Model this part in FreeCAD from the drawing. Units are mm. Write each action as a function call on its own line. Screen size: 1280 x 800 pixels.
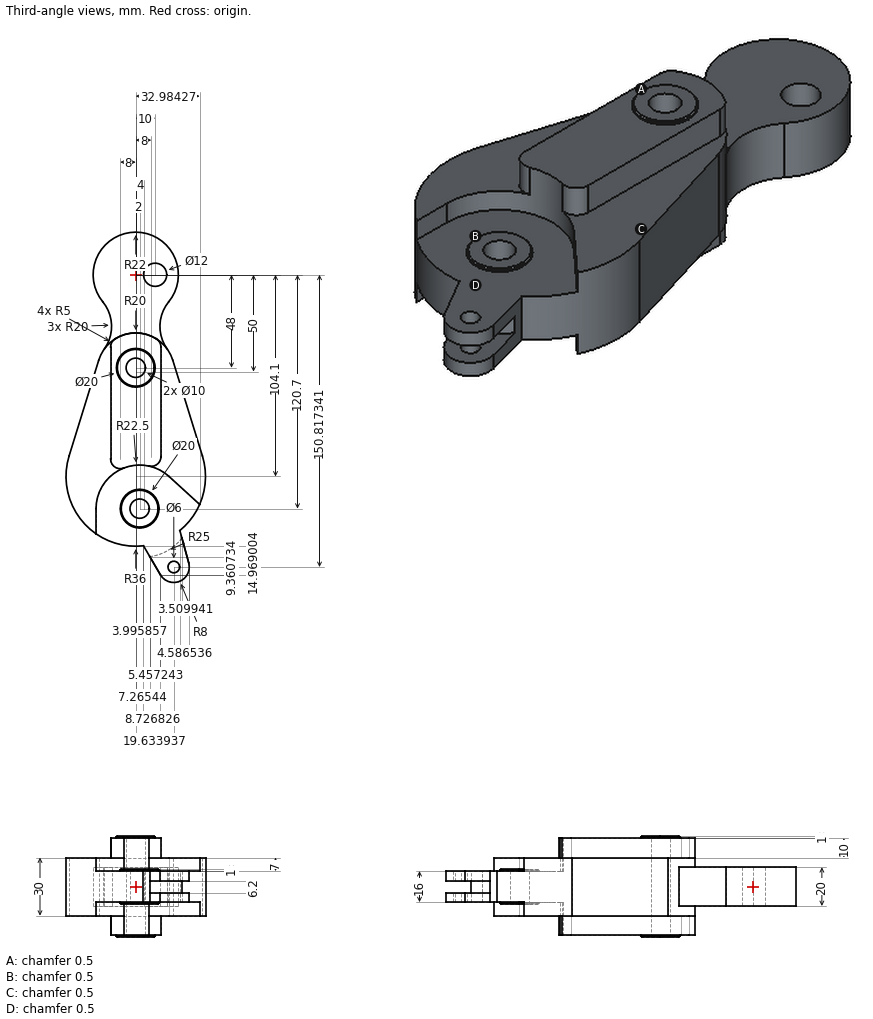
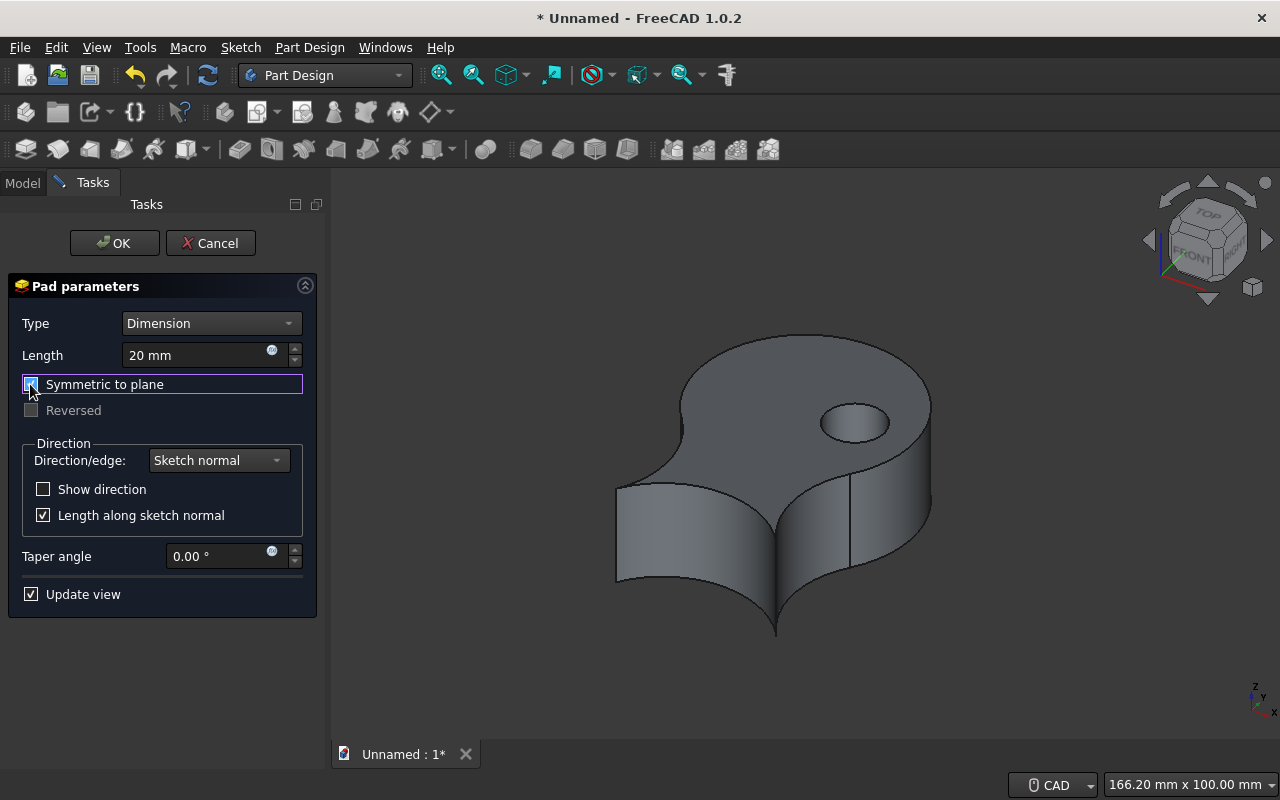
click(115, 243)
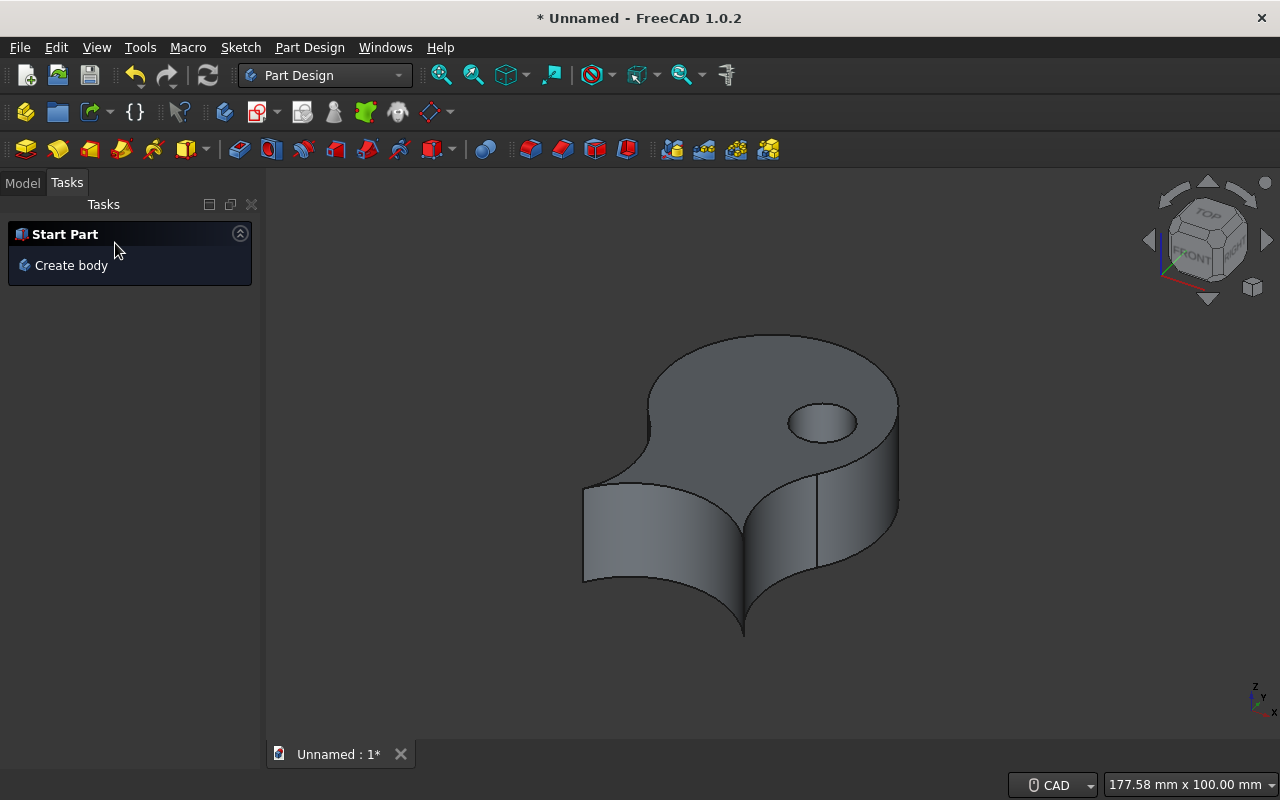
click(258, 112)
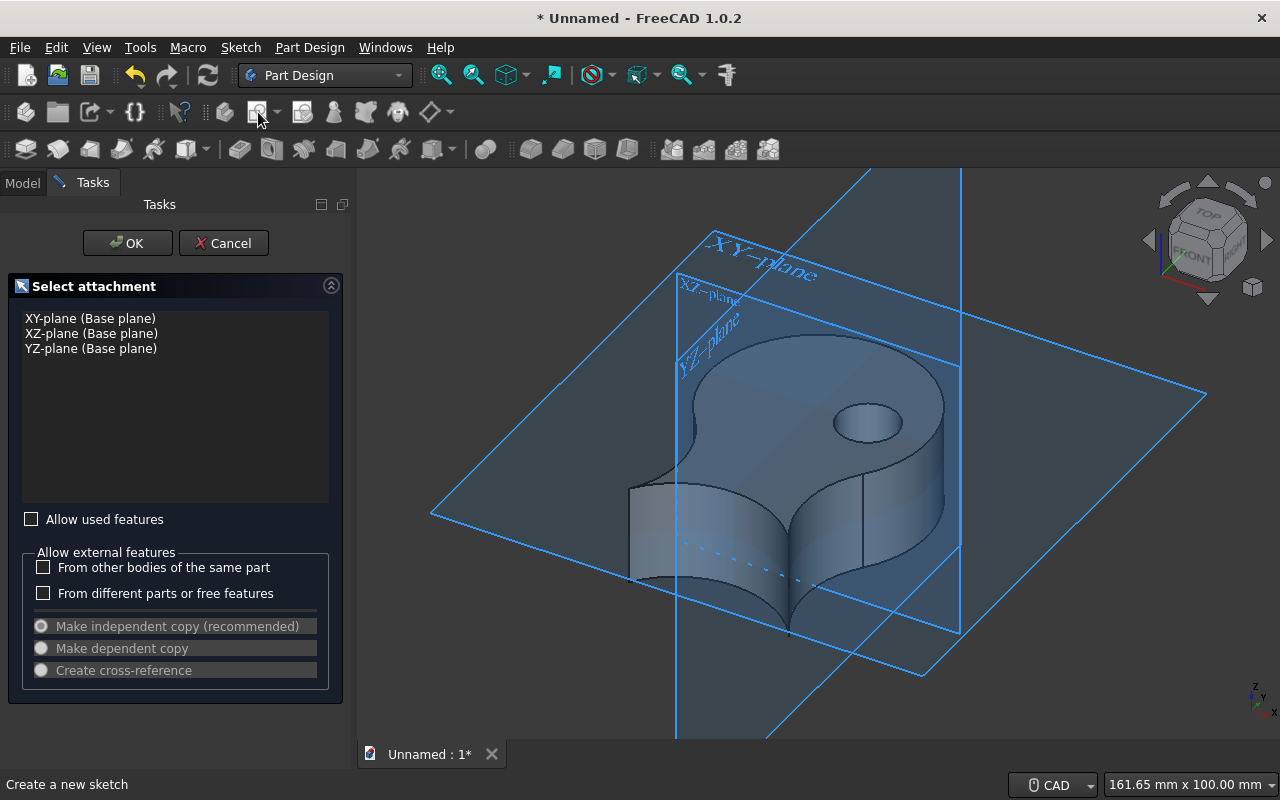
click(82, 318)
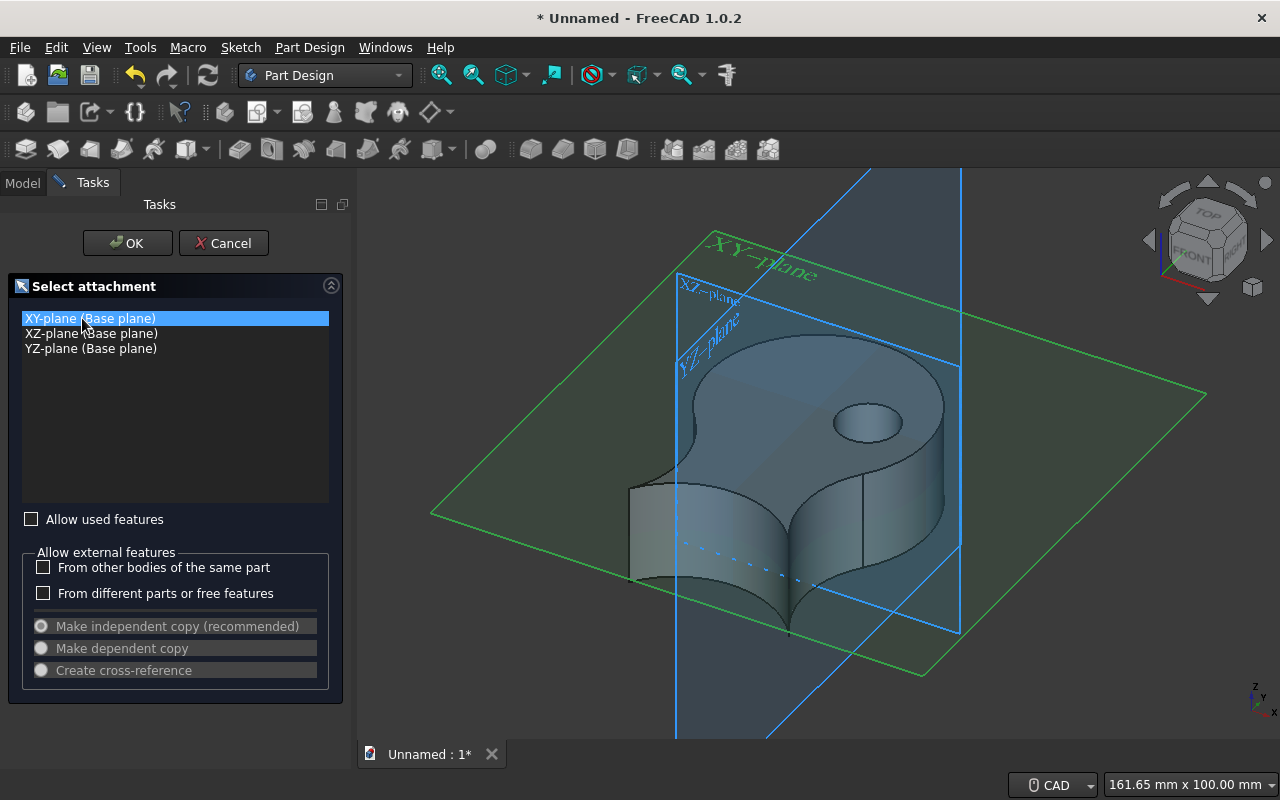
click(128, 243)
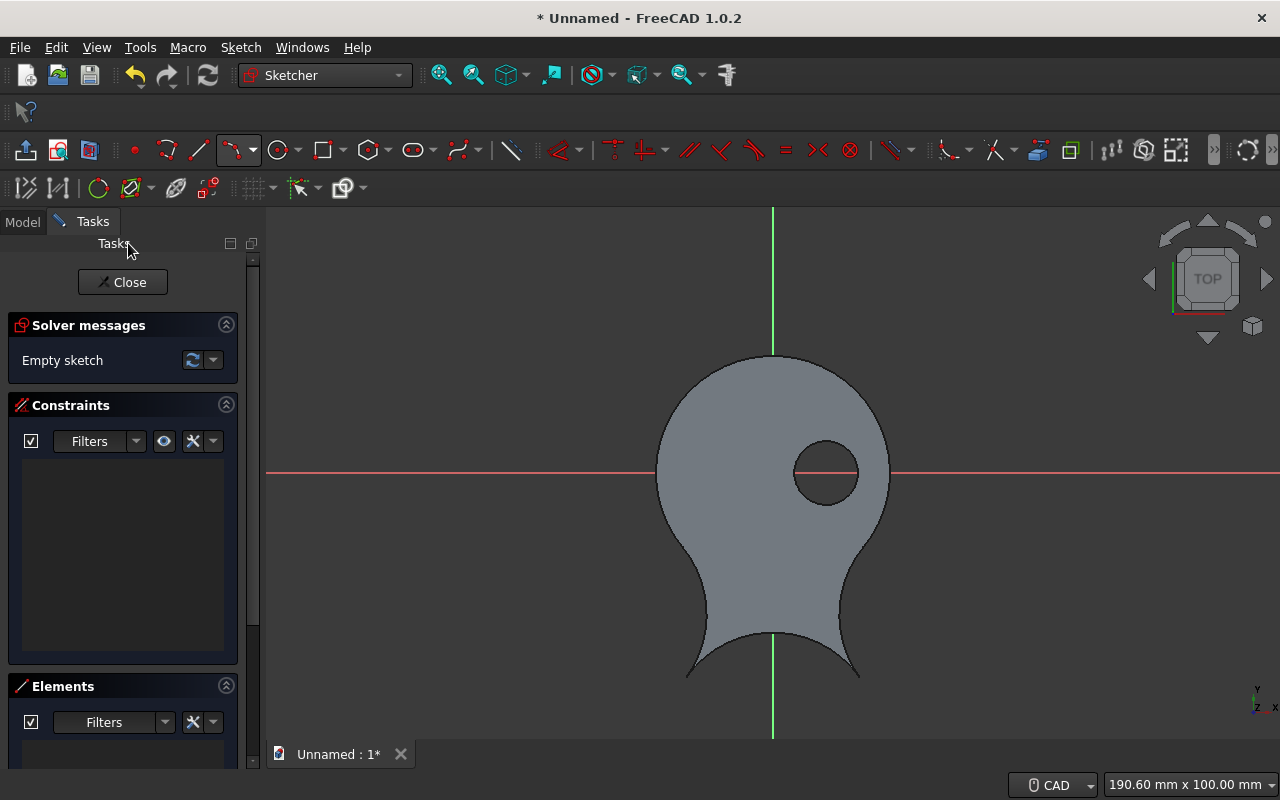
click(90, 150)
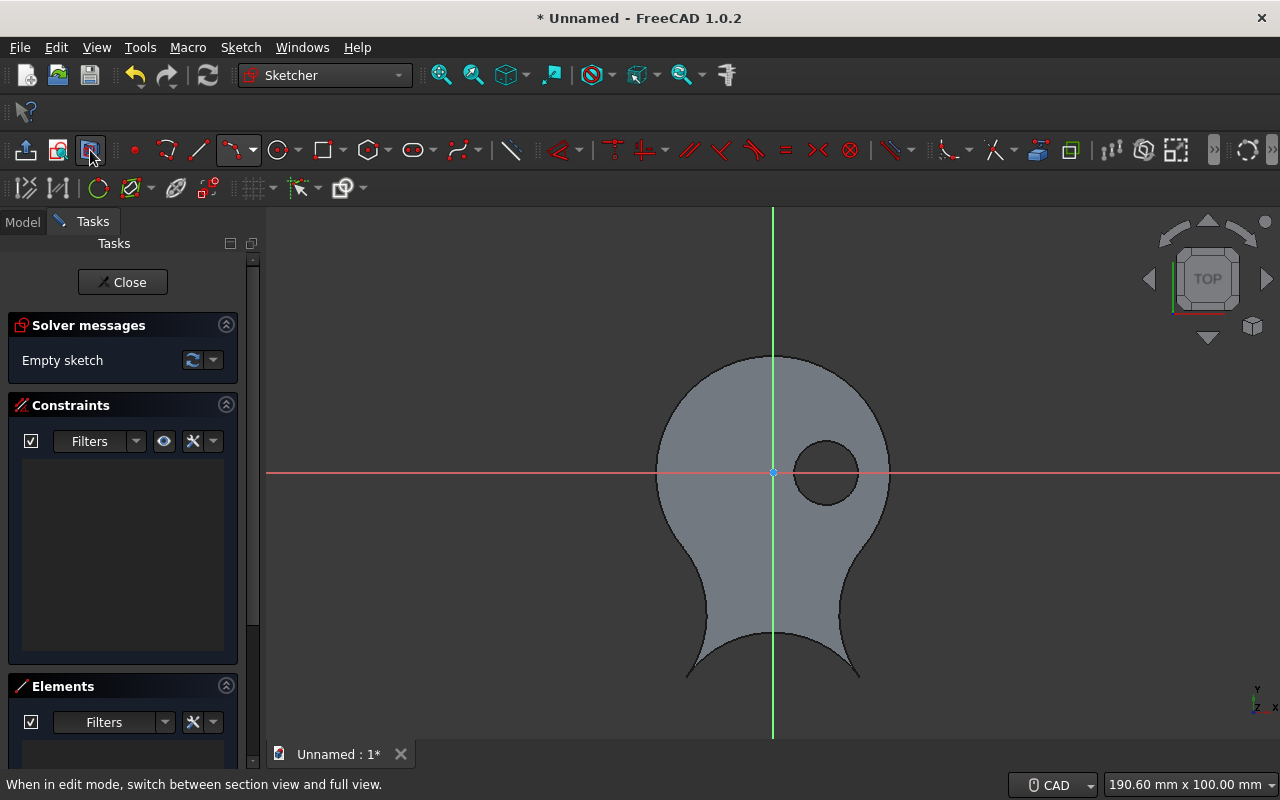
scroll(649, 235, down, 4)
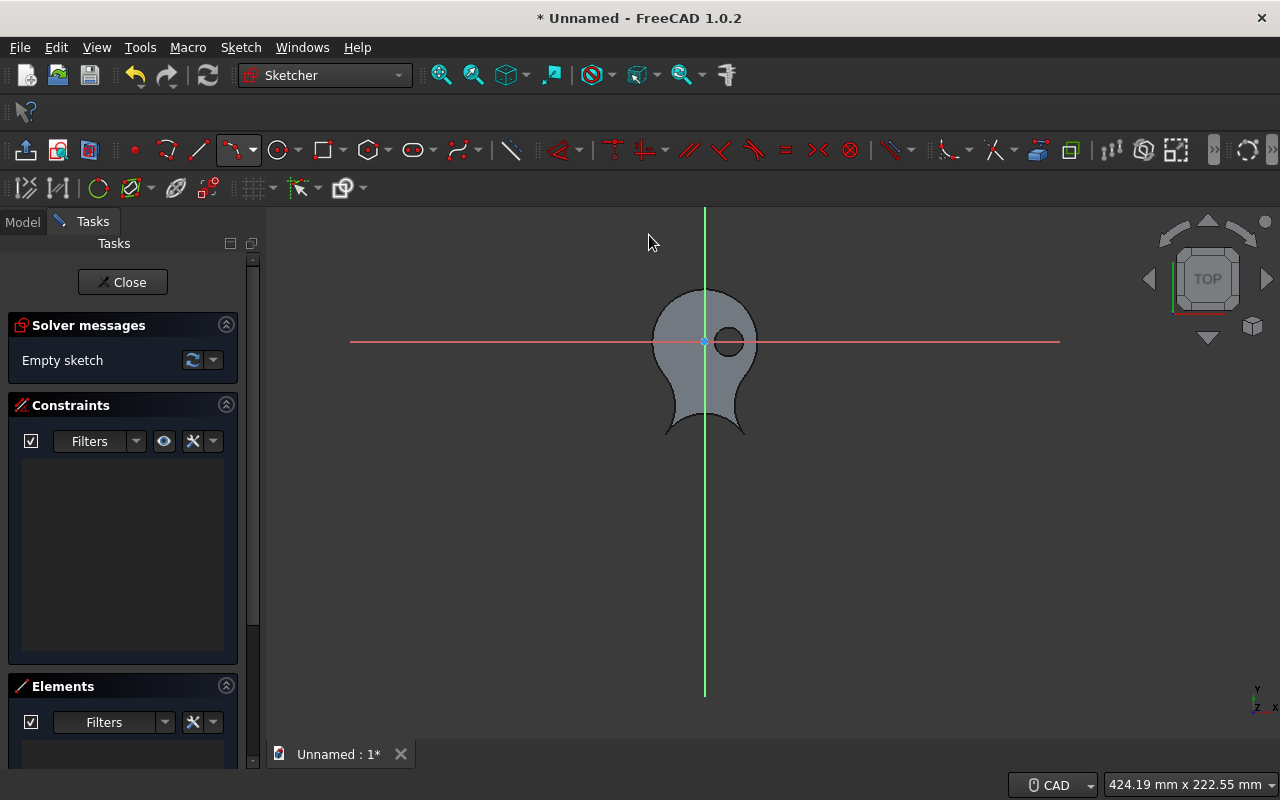
click(200, 150)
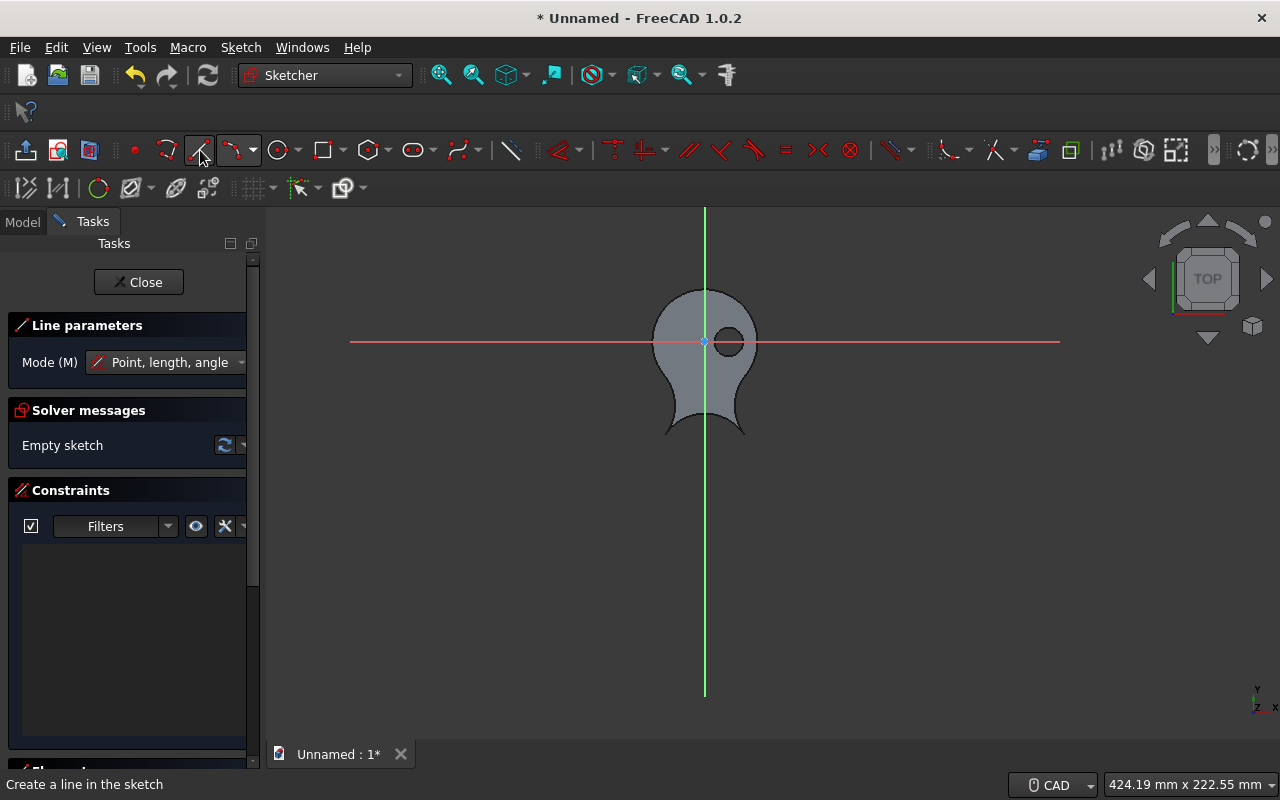
click(659, 447)
click(623, 565)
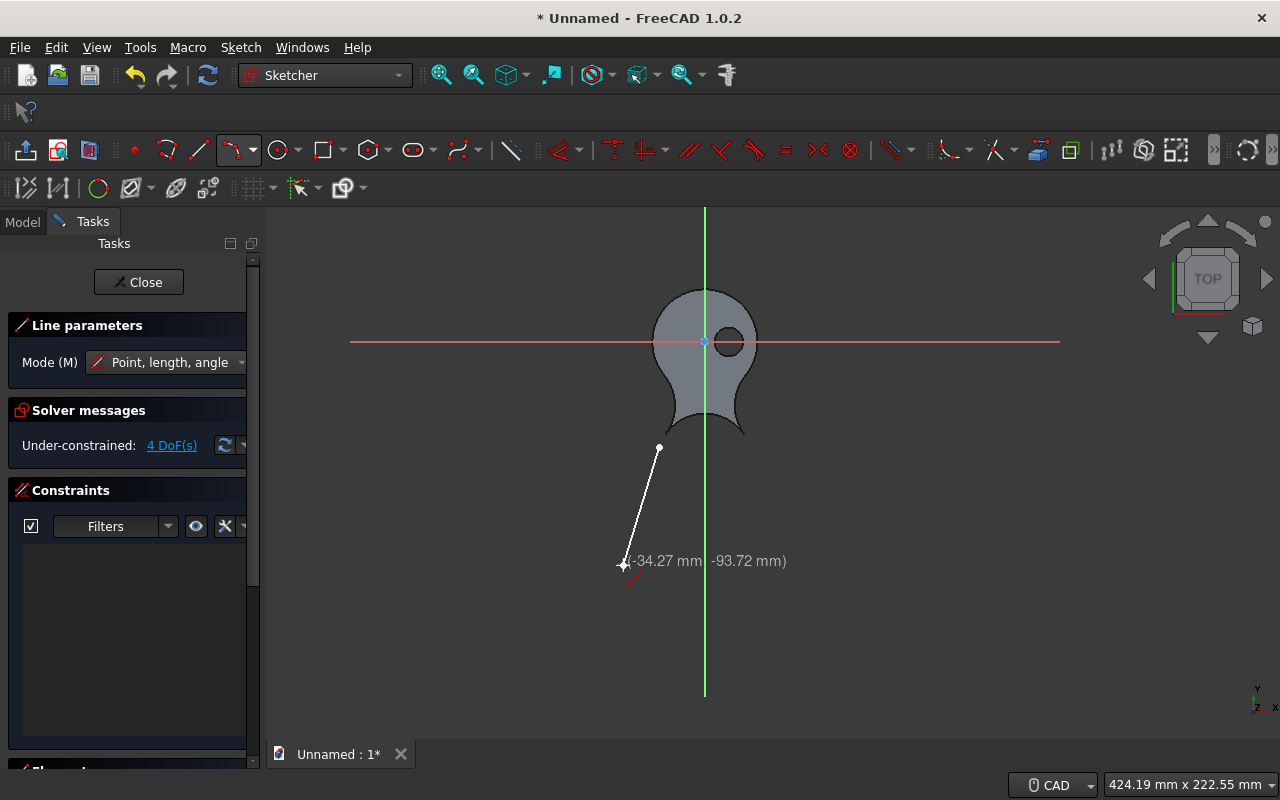
click(787, 565)
click(751, 447)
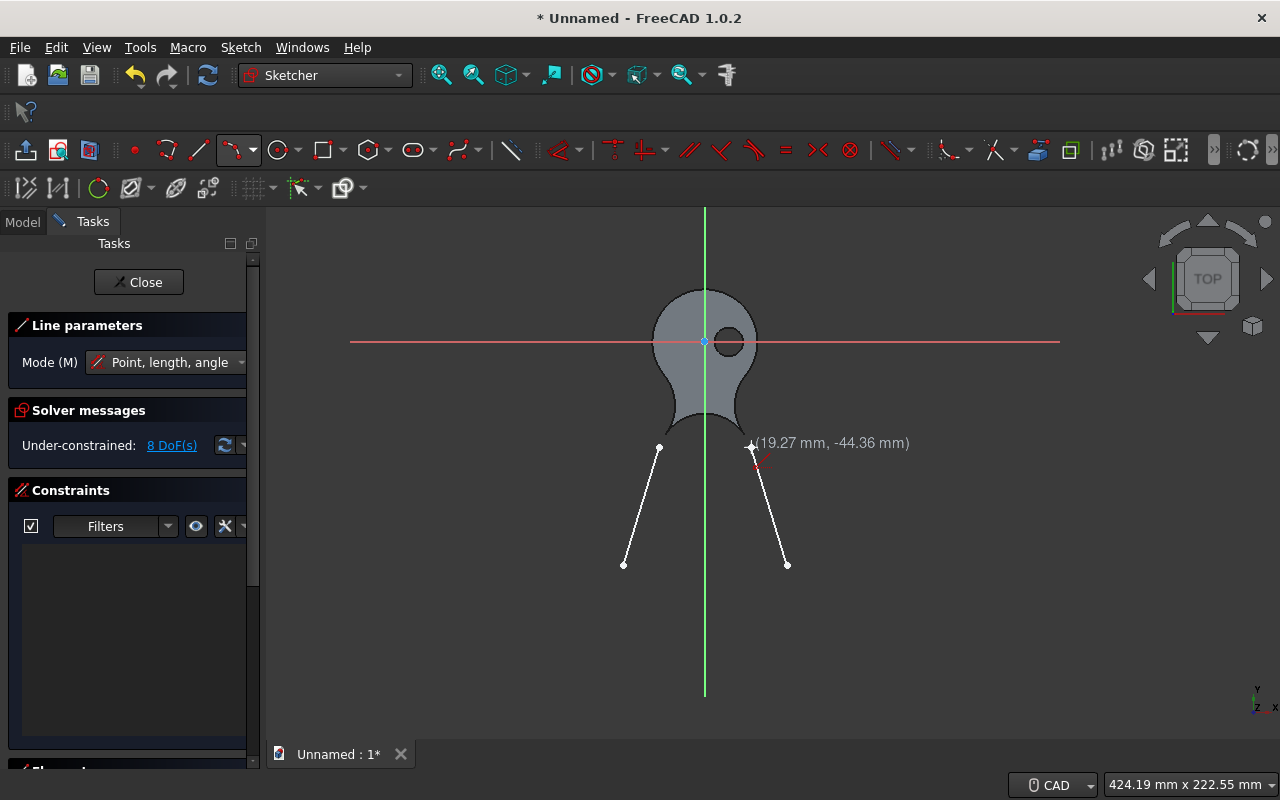
click(232, 150)